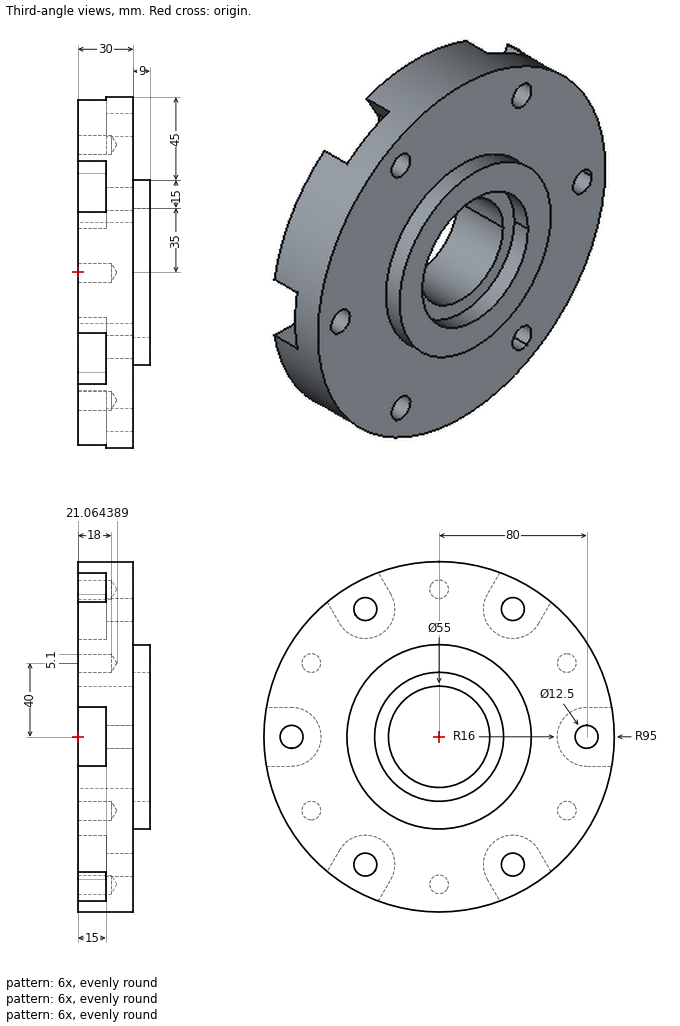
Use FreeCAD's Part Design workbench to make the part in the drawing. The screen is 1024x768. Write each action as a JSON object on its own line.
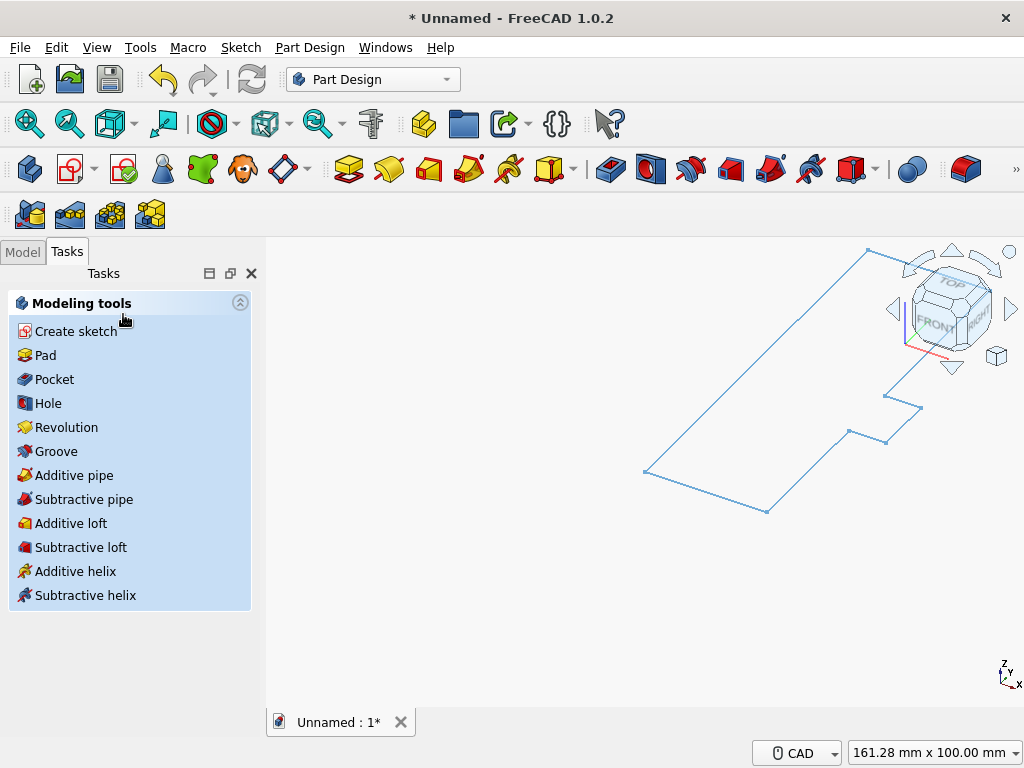
{"action": "left_click", "coordinate": [390, 170]}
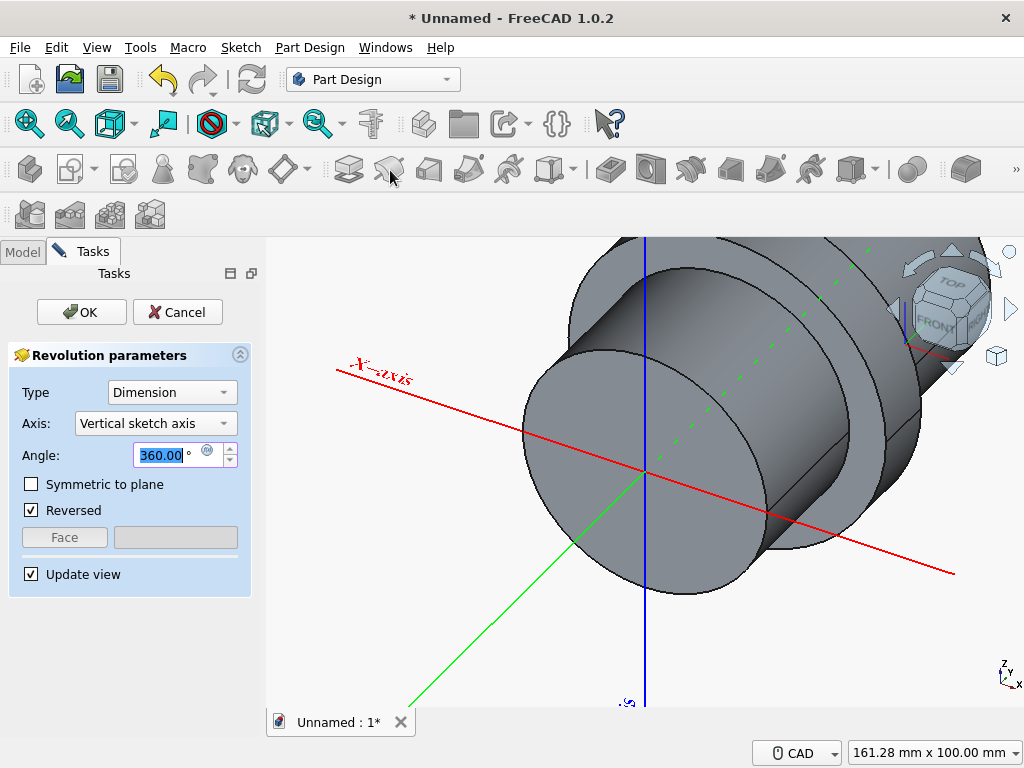
{"action": "left_click", "coordinate": [156, 424]}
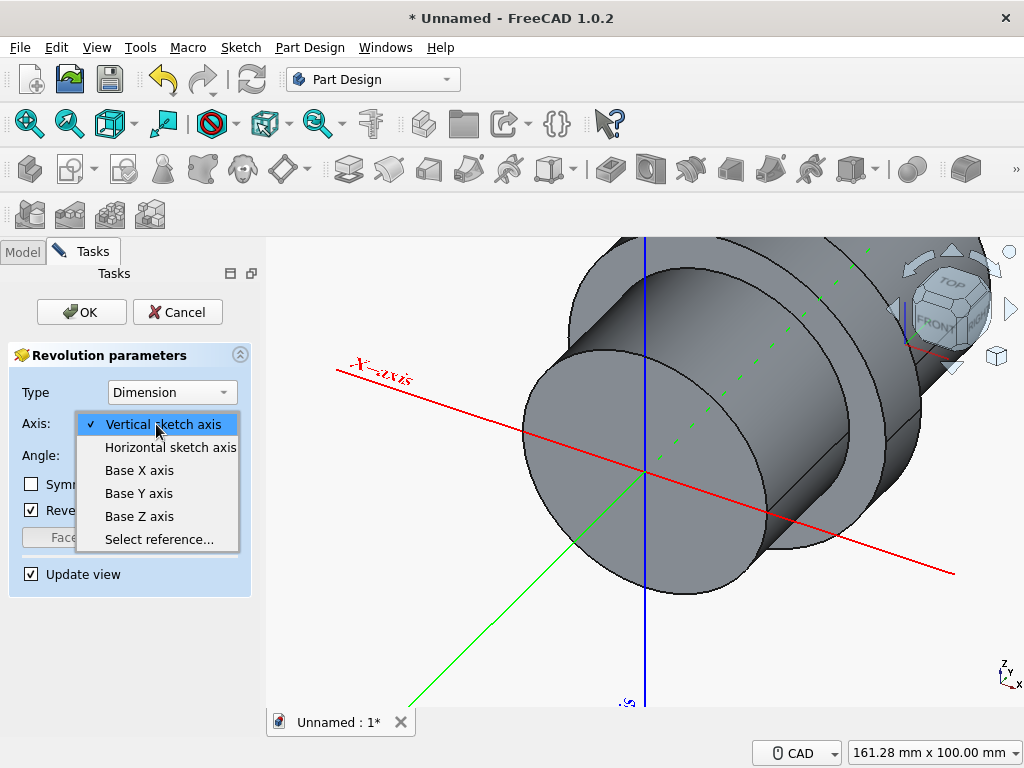
{"action": "left_click", "coordinate": [156, 448]}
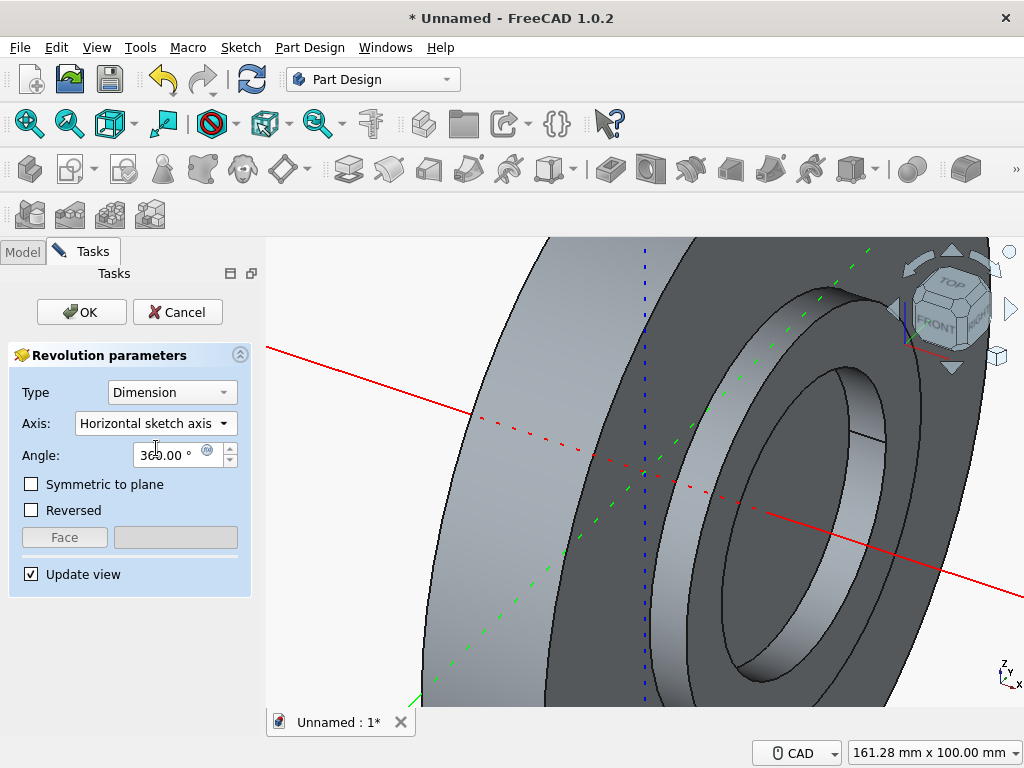
{"action": "left_click", "coordinate": [82, 312]}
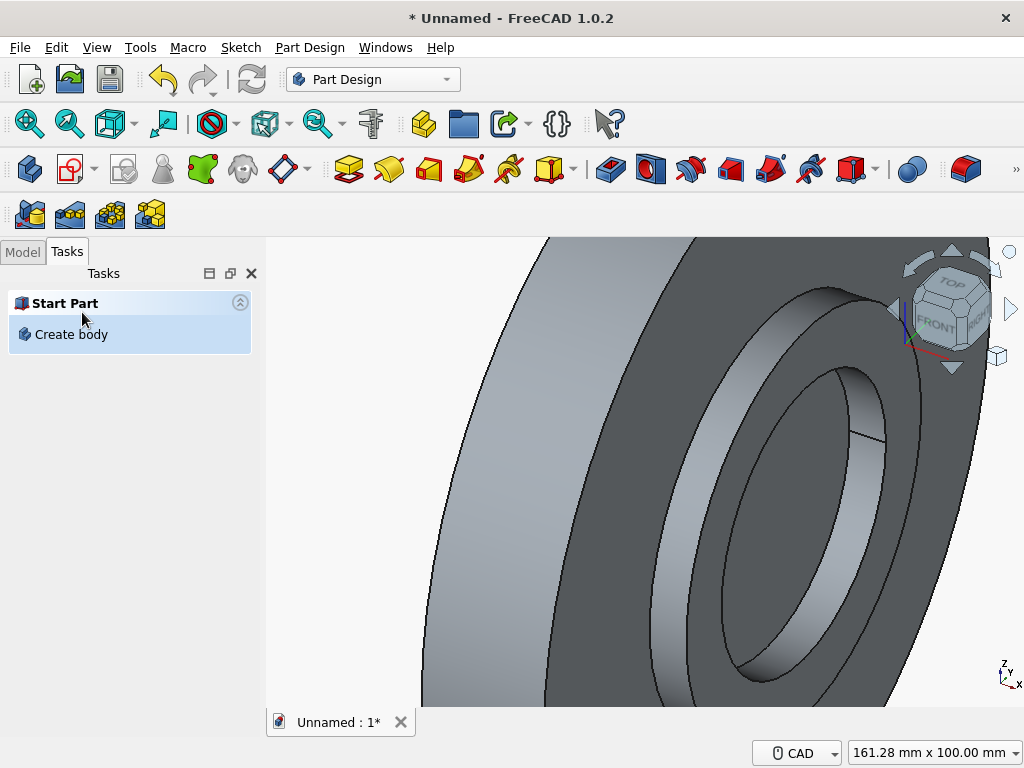
{"action": "key", "text": "v f"}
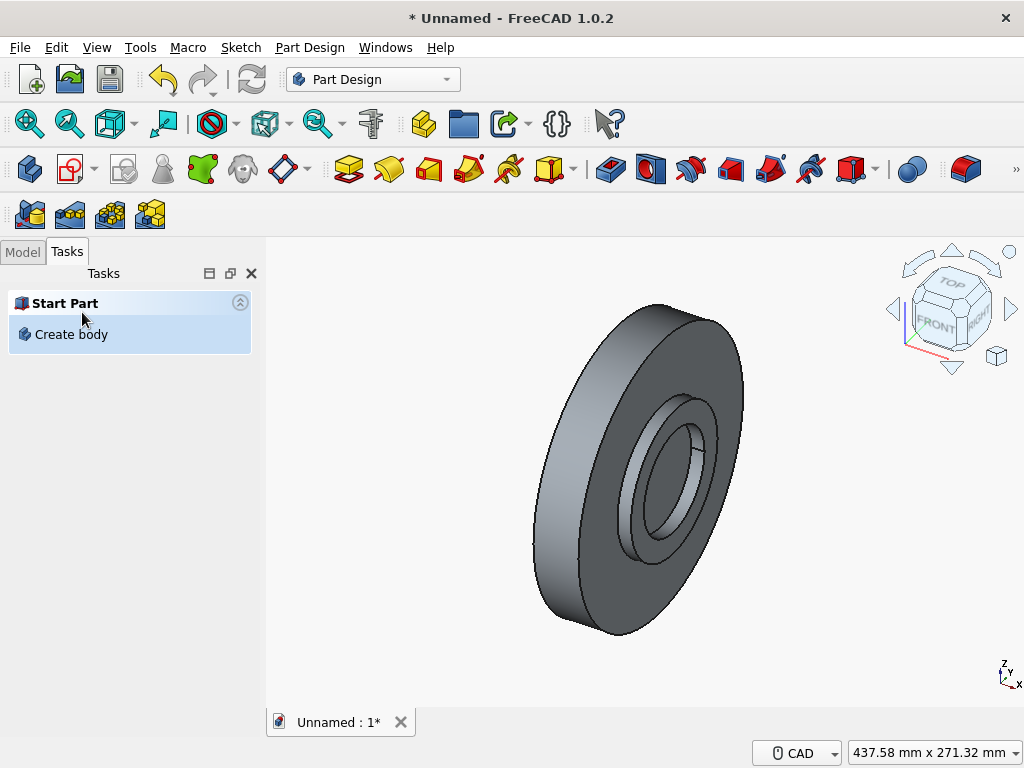
{"action": "left_click", "coordinate": [70, 170]}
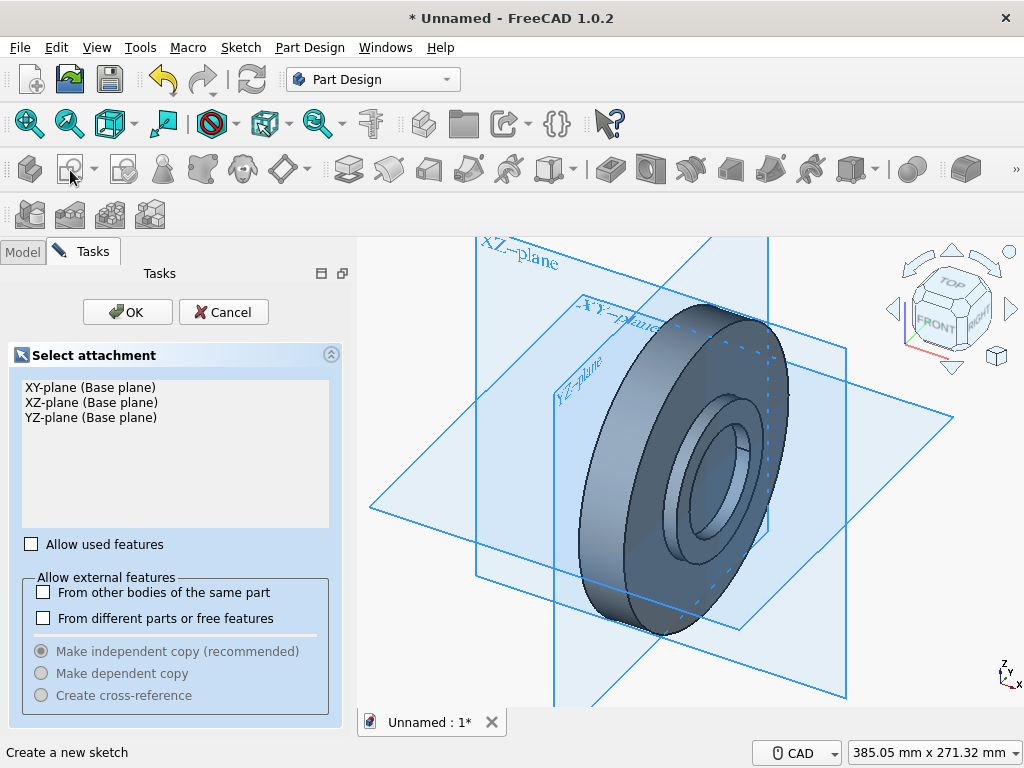
{"action": "left_click", "coordinate": [82, 418]}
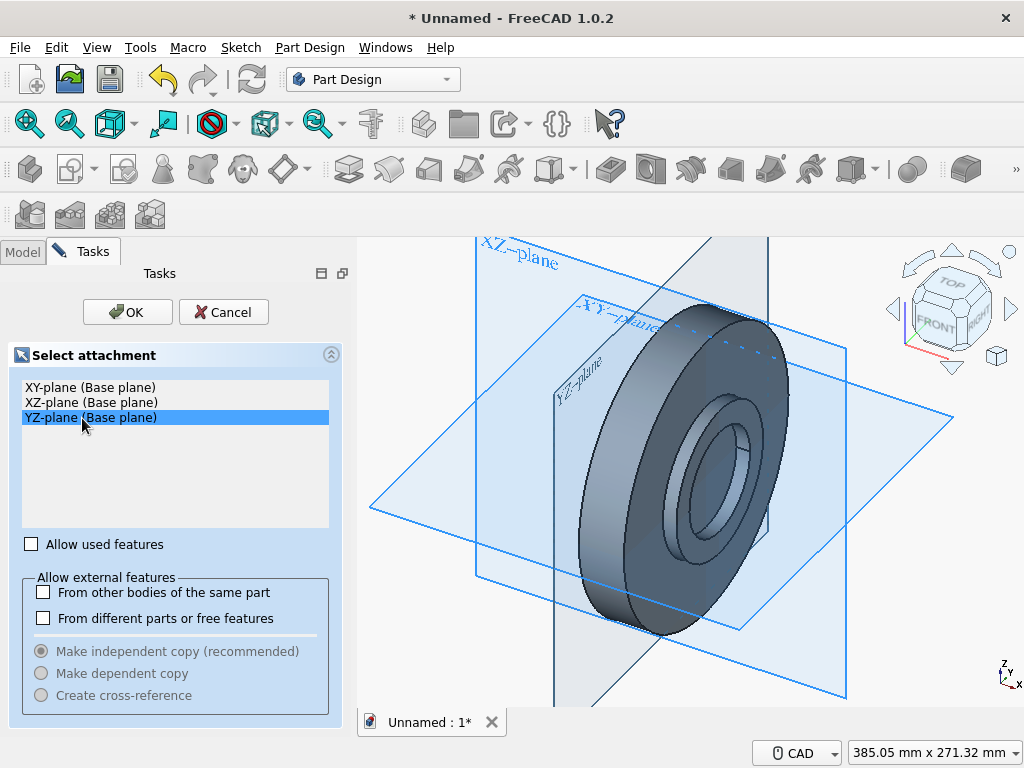
{"action": "left_click", "coordinate": [128, 312]}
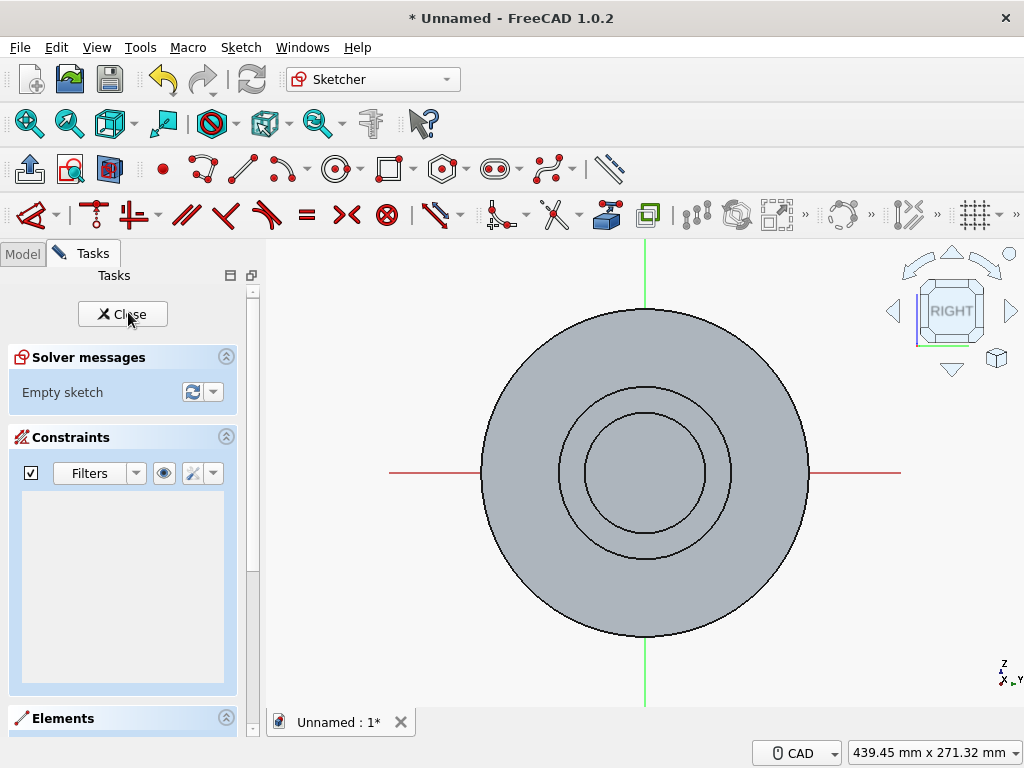
{"action": "left_click", "coordinate": [110, 170]}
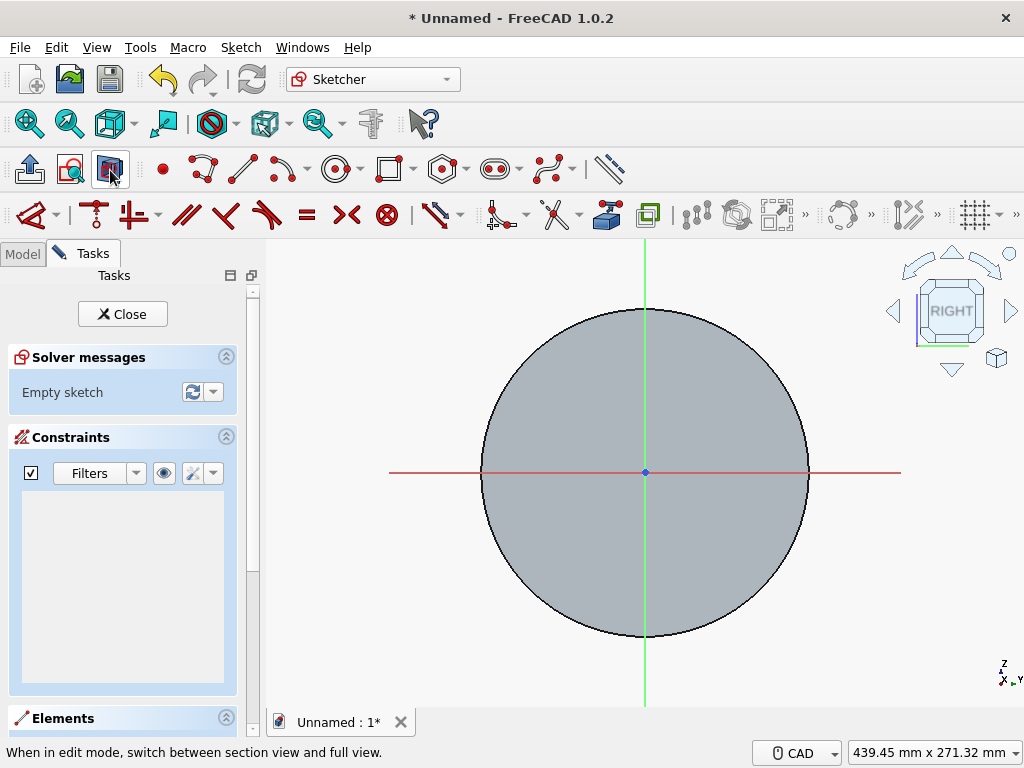
{"action": "scroll", "coordinate": [800, 473], "scroll_direction": "up", "scroll_amount": 13}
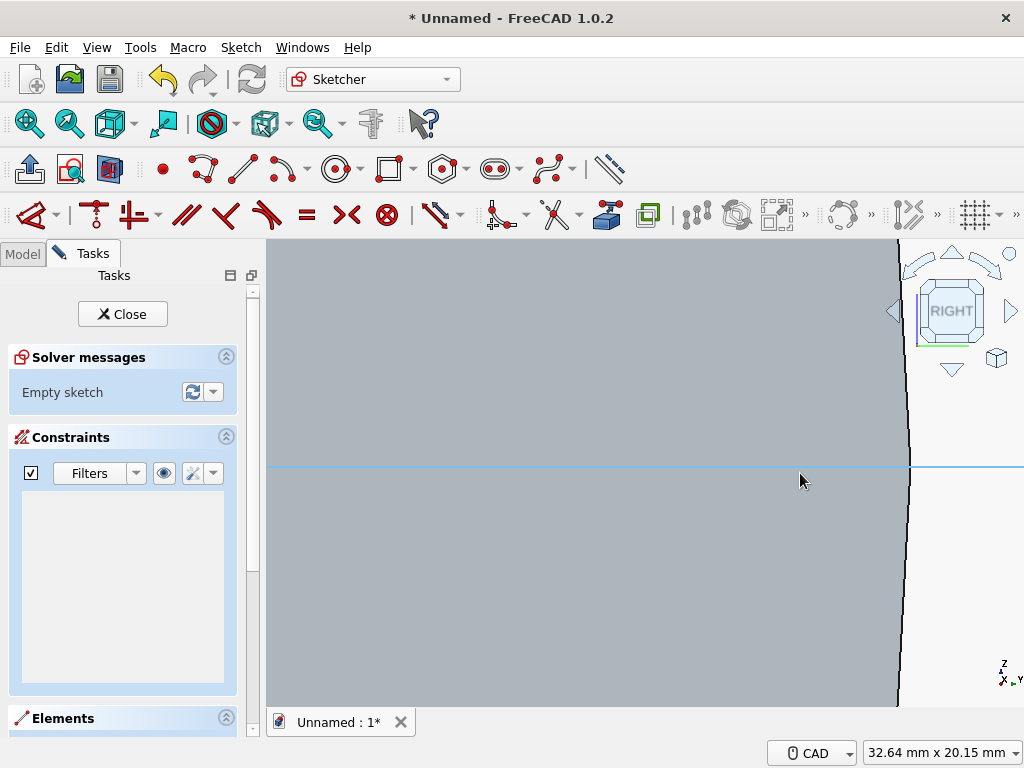
{"action": "left_click", "coordinate": [336, 170]}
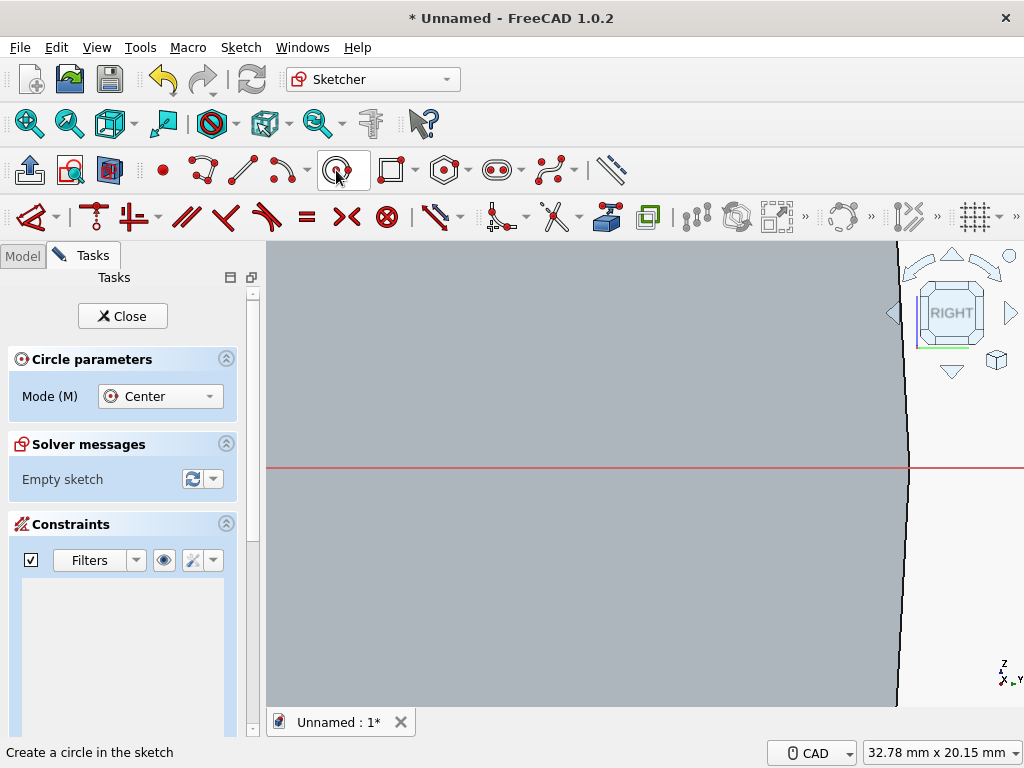
{"action": "left_click", "coordinate": [563, 468]}
{"action": "mouse_move", "coordinate": [665, 366]}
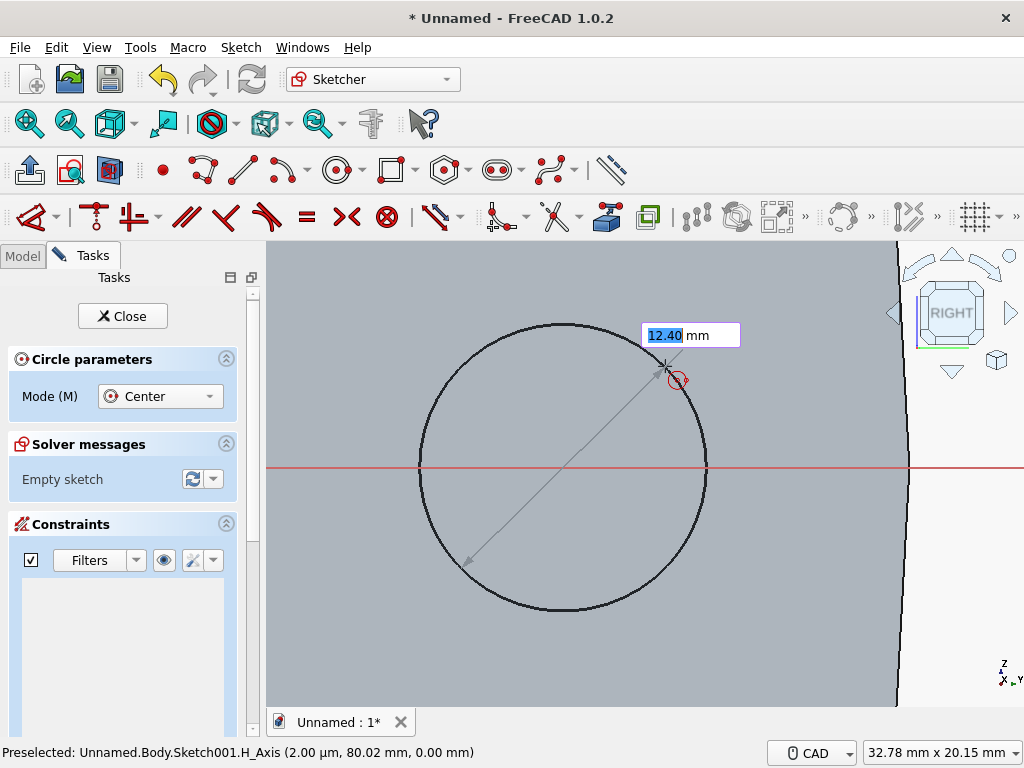
{"action": "type", "text": "12.5"}
{"action": "key", "text": "Return"}
{"action": "key", "text": "Escape"}